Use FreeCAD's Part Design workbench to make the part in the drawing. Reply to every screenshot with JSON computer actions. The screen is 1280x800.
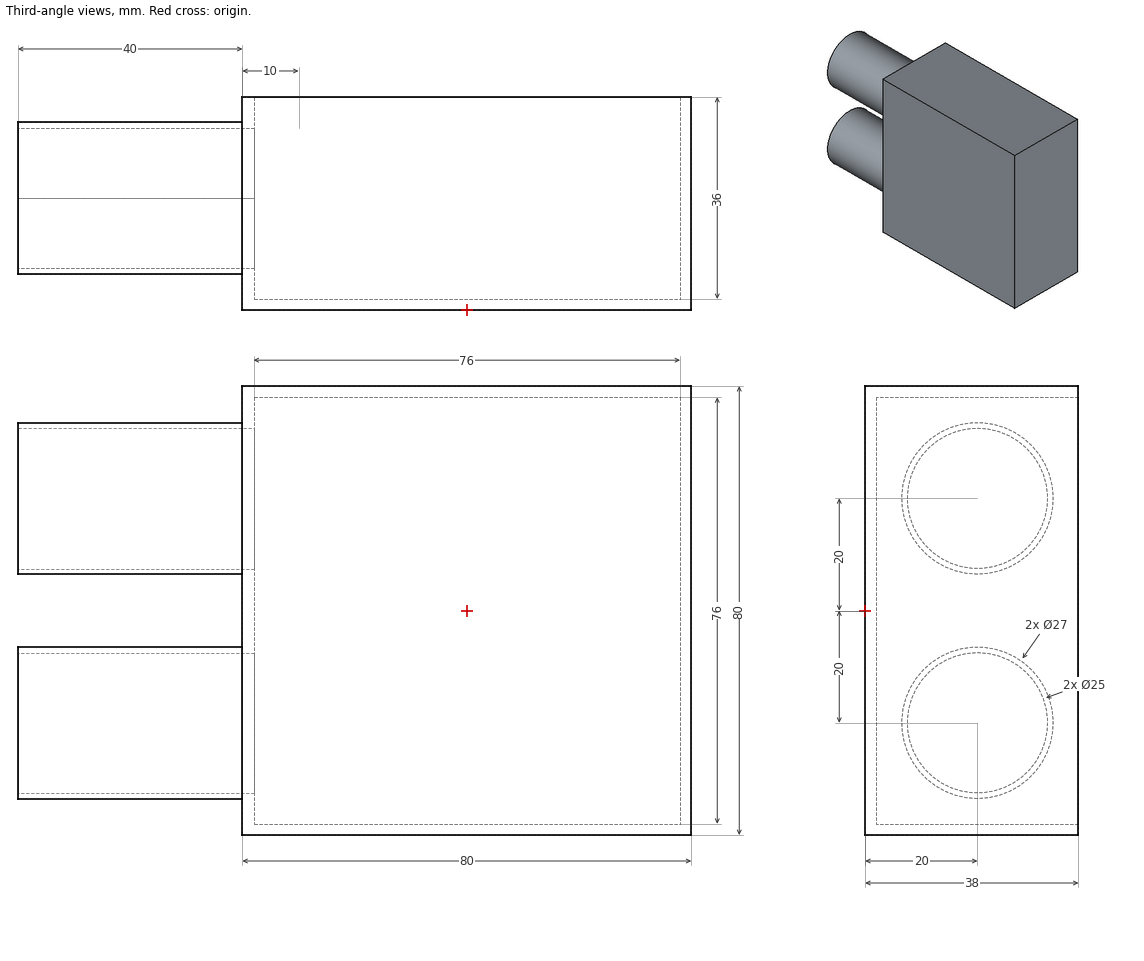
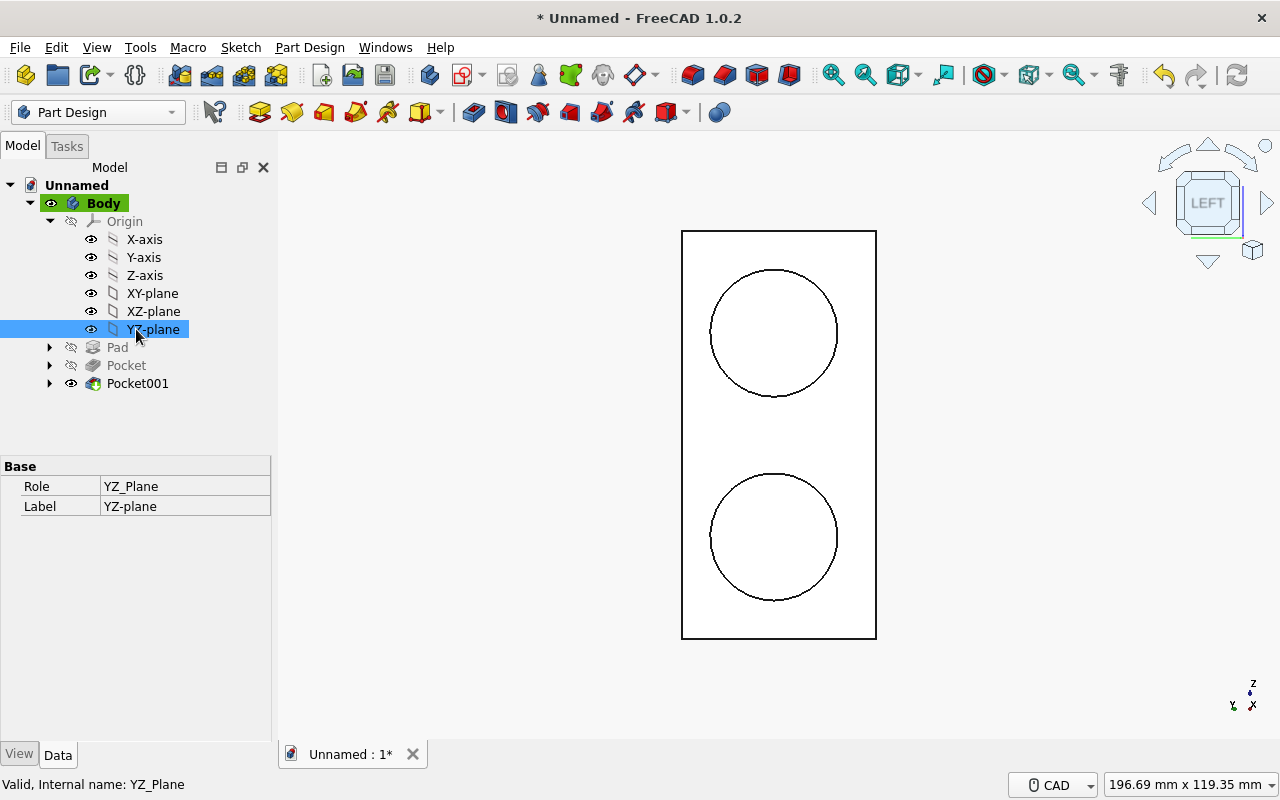
{"action": "left_click", "coordinate": [636, 76]}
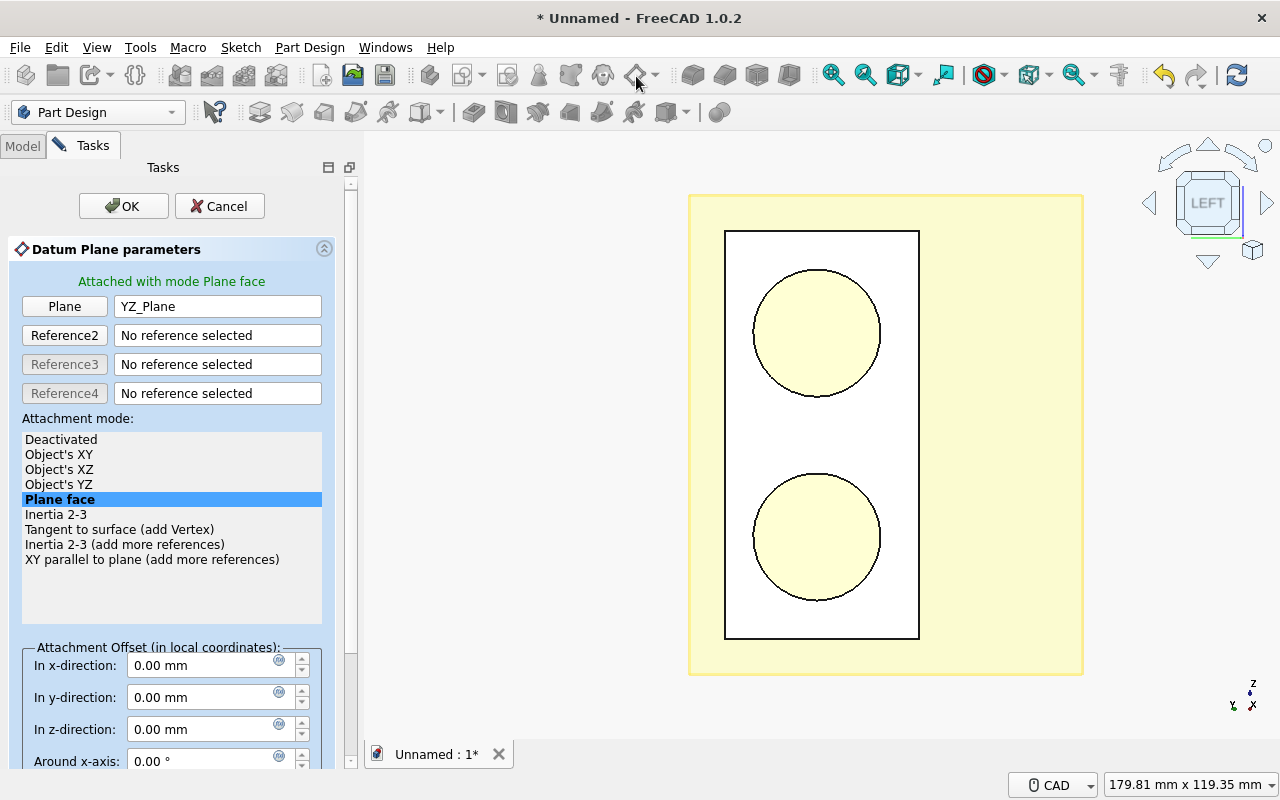
{"action": "triple_click", "coordinate": [210, 729]}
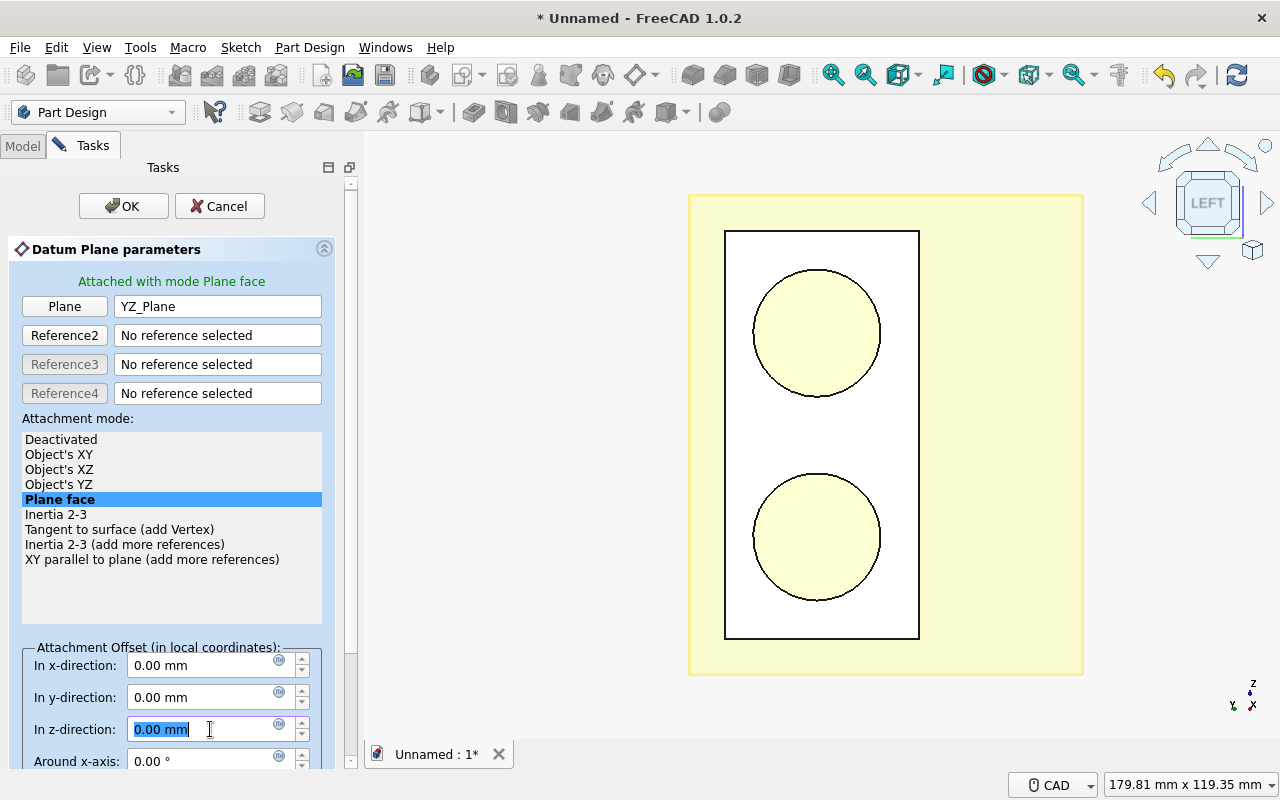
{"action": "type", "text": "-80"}
{"action": "key", "text": "Tab"}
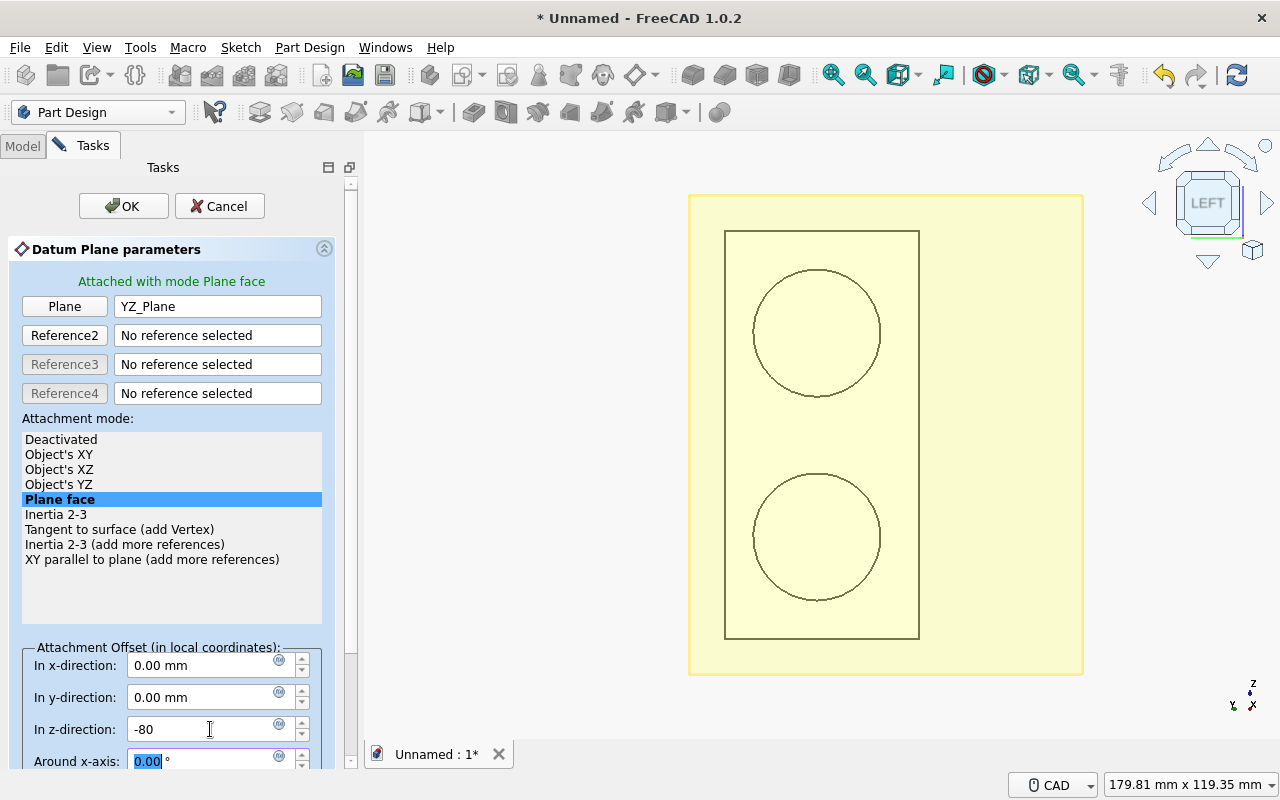
{"action": "left_click", "coordinate": [124, 206]}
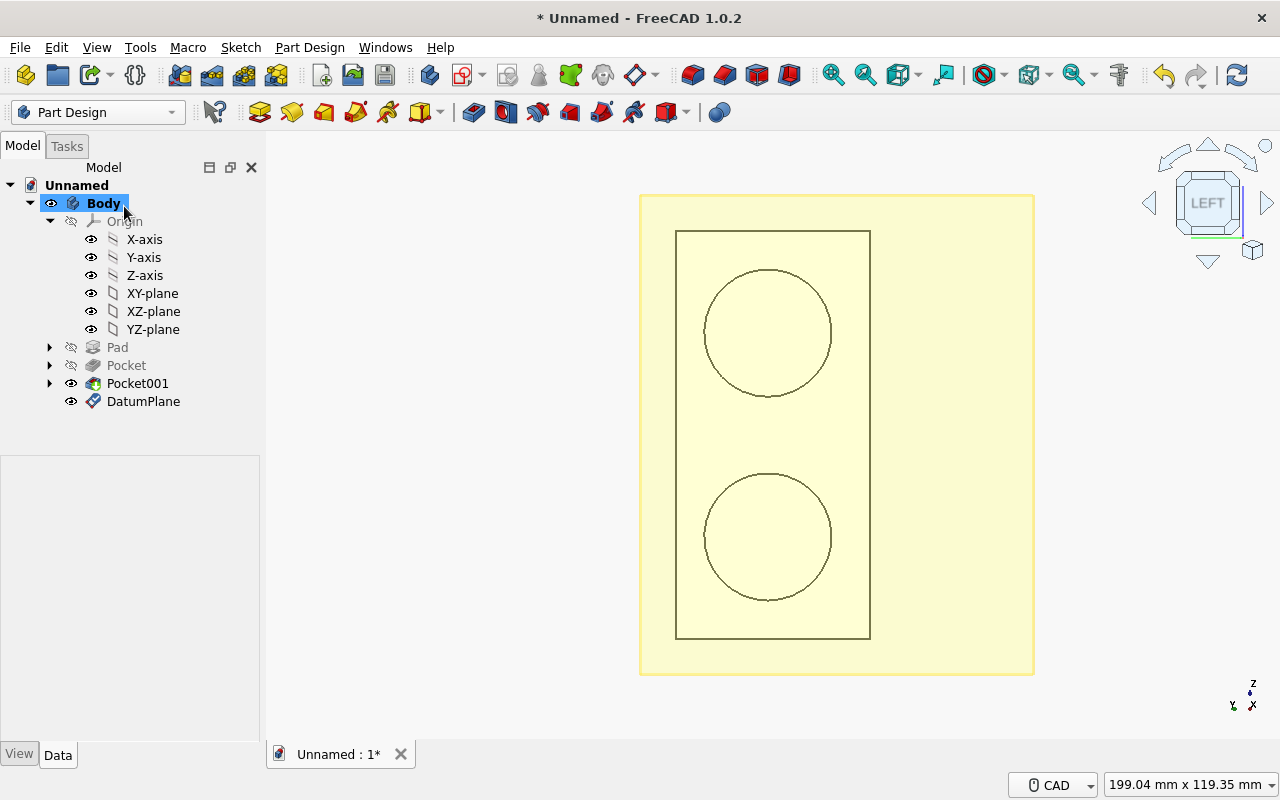
{"action": "left_click", "coordinate": [116, 401]}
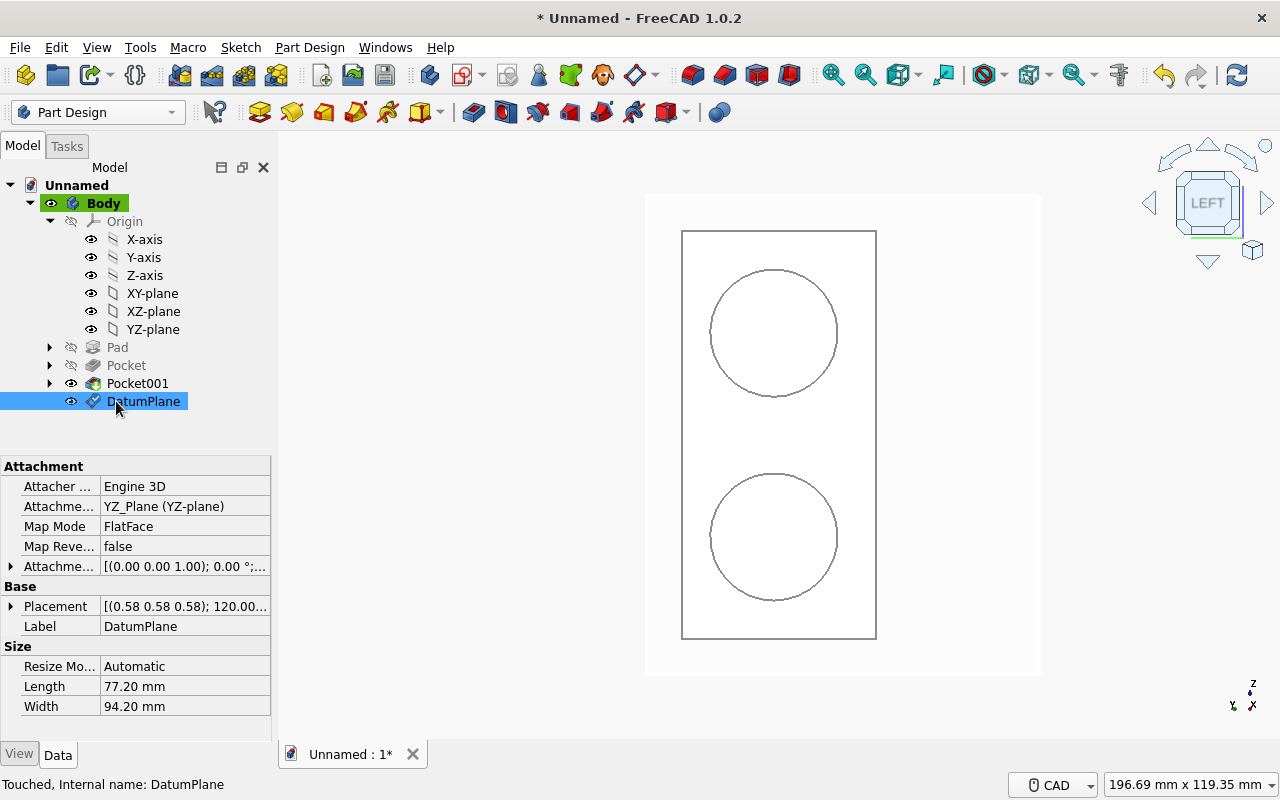
{"action": "left_click", "coordinate": [462, 76]}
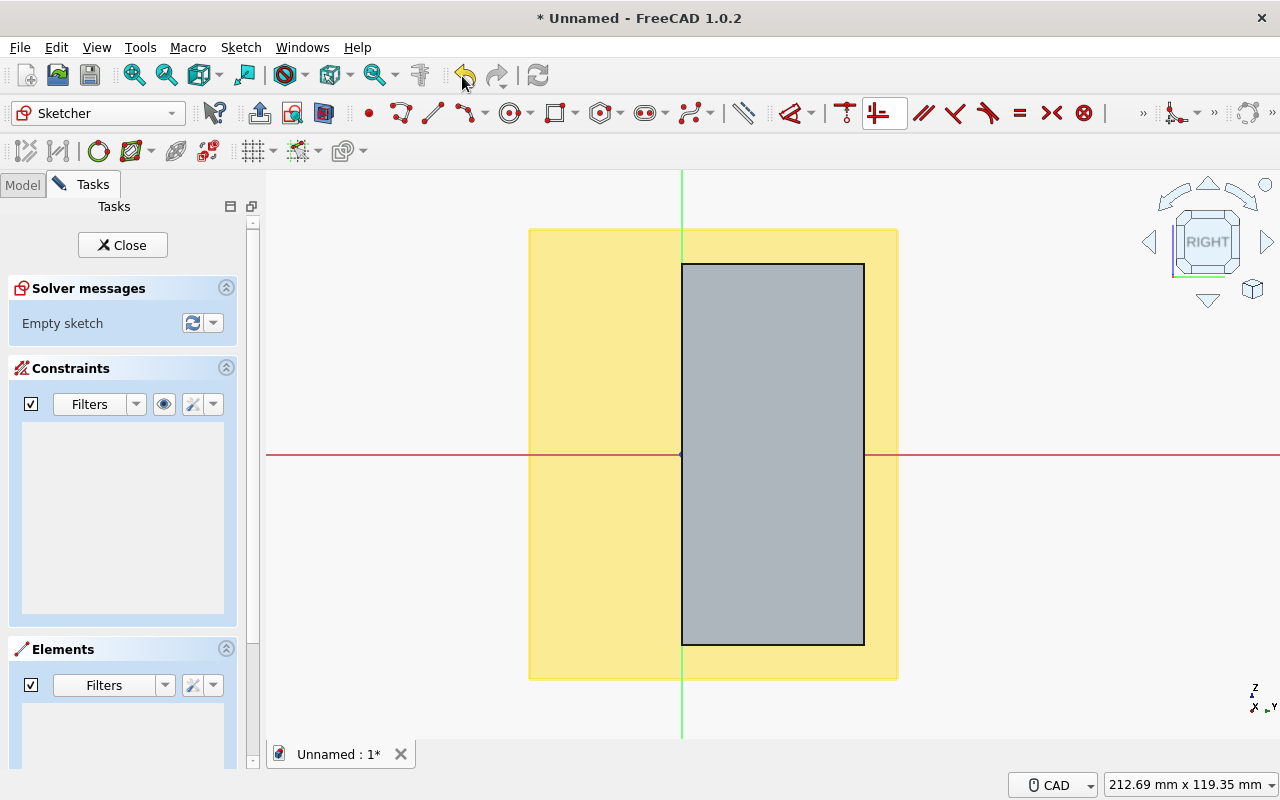
{"action": "left_click", "coordinate": [324, 114]}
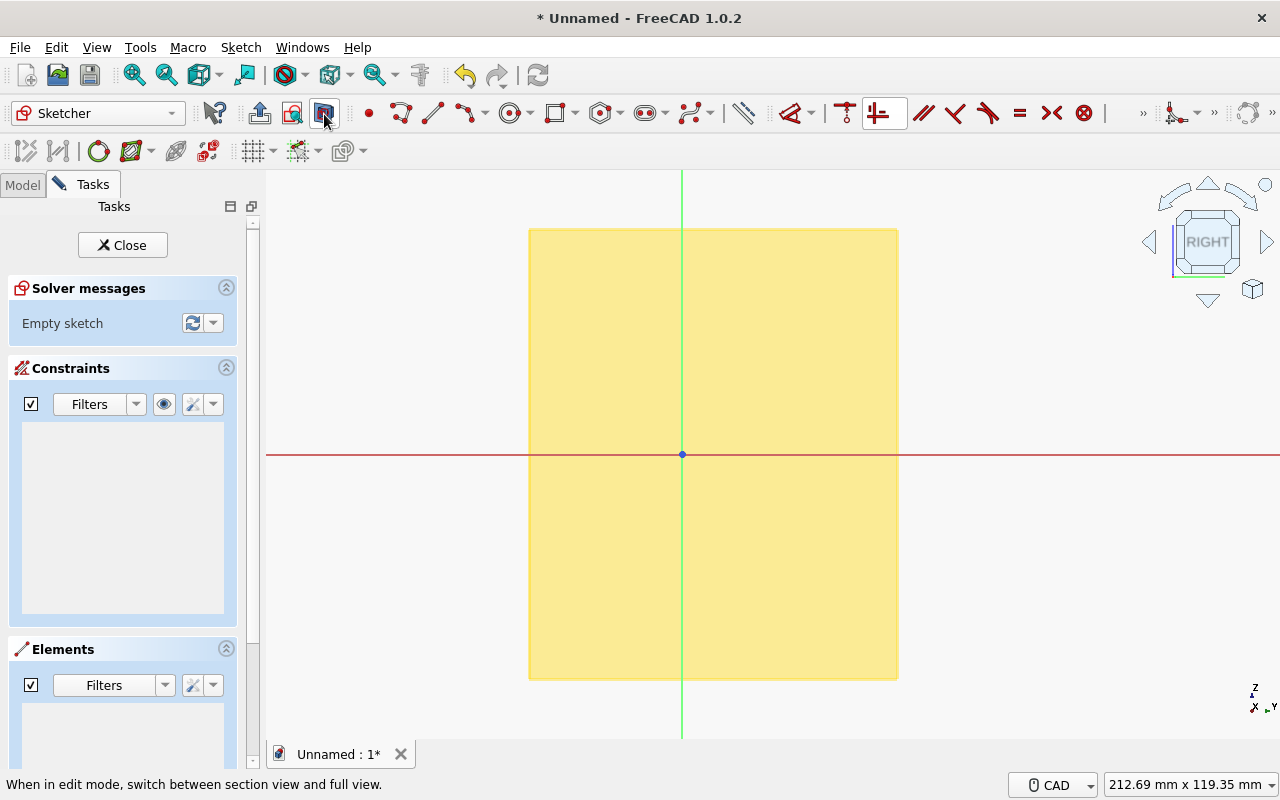
{"action": "left_click", "coordinate": [510, 114]}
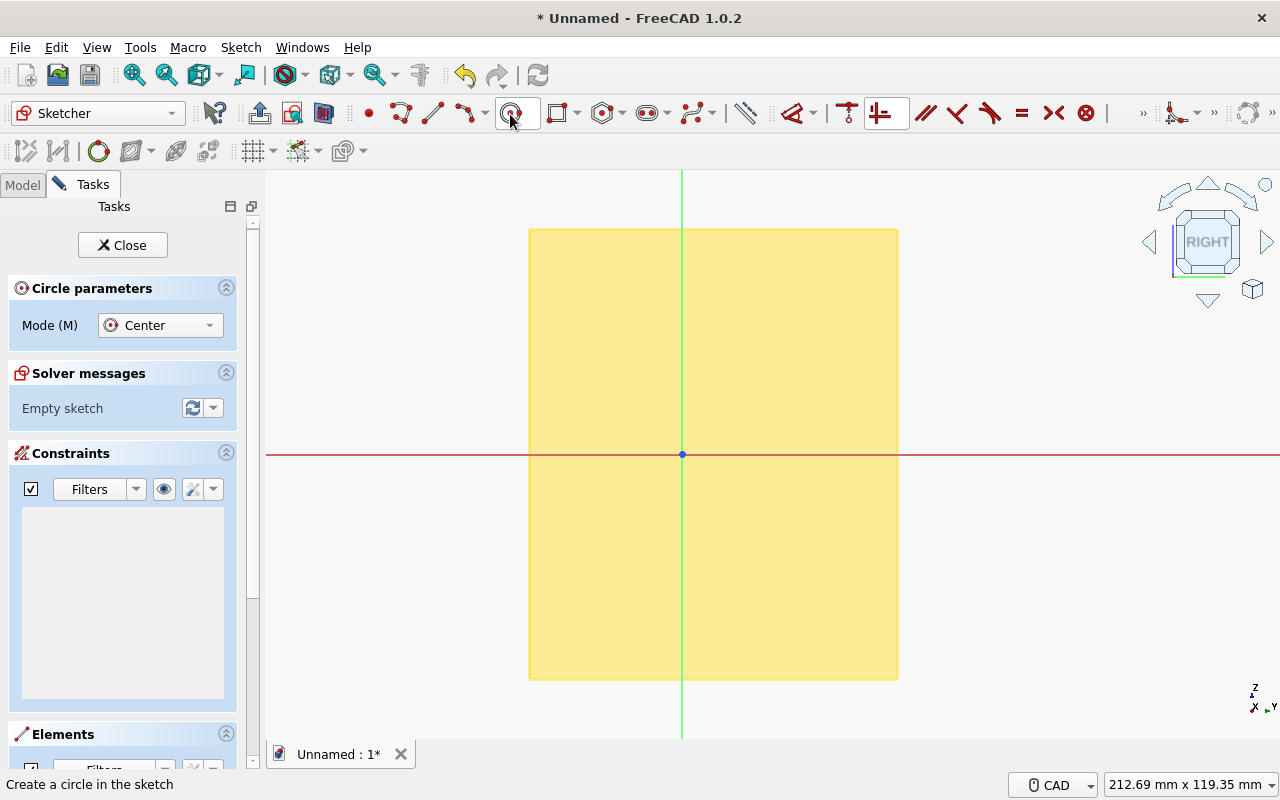
{"action": "left_click", "coordinate": [778, 550]}
{"action": "mouse_move", "coordinate": [823, 504]}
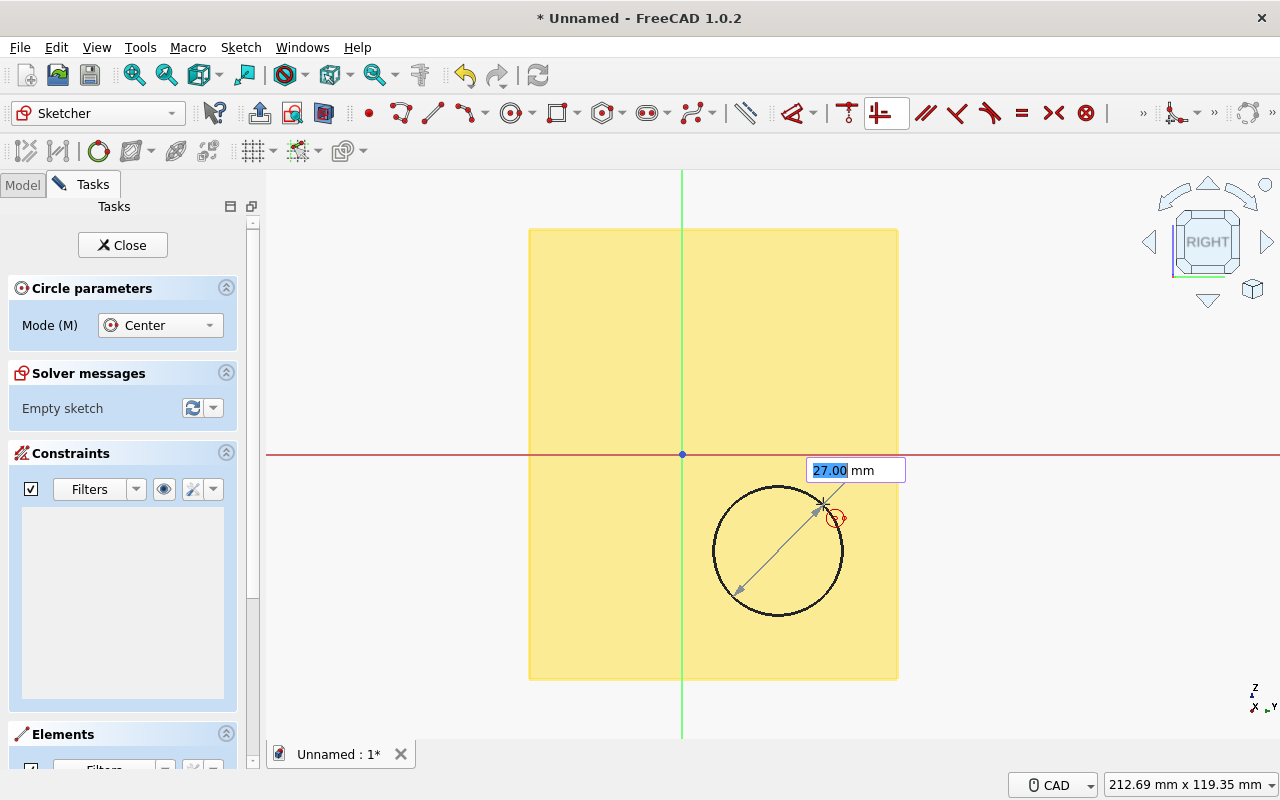
{"action": "type", "text": "27"}
{"action": "key", "text": "Return"}